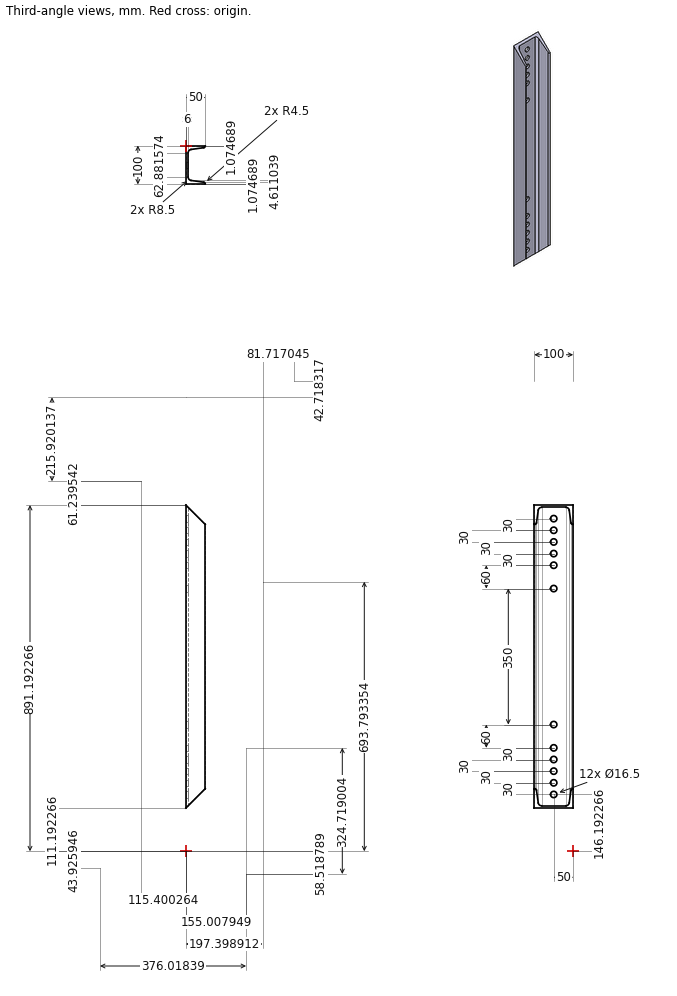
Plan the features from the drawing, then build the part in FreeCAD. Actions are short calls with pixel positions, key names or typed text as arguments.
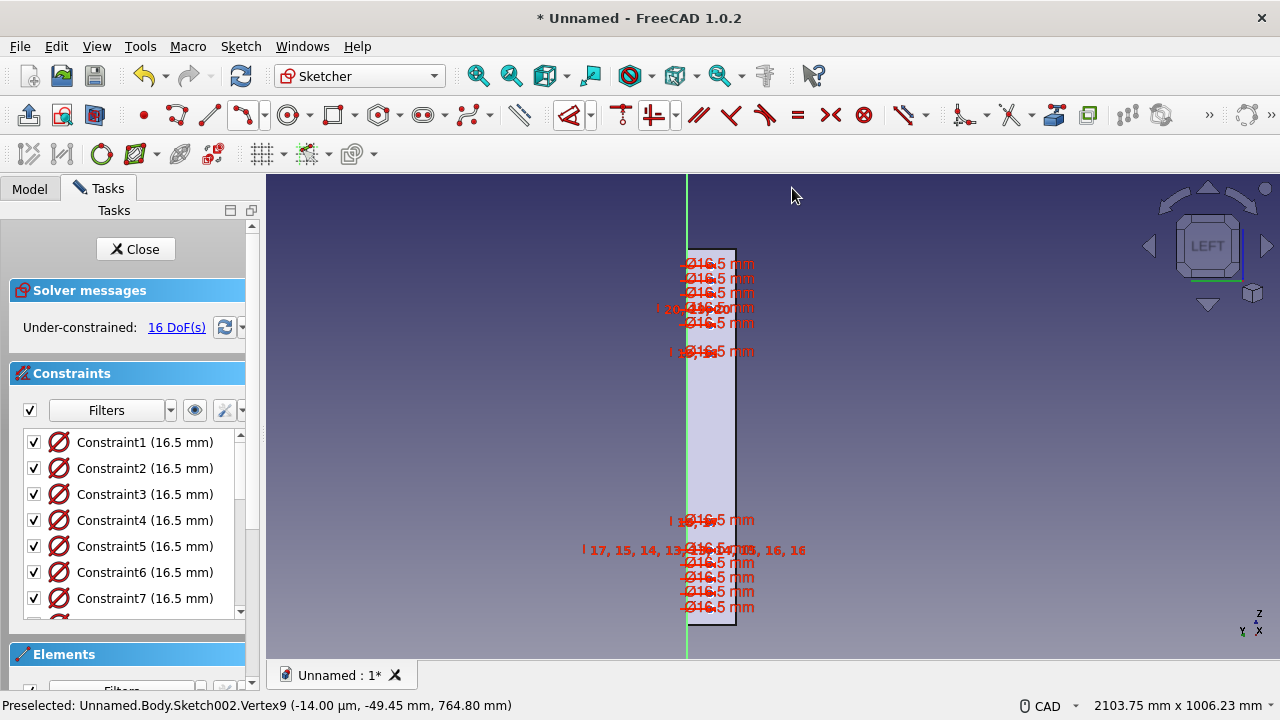
scroll(711, 310, up, 4)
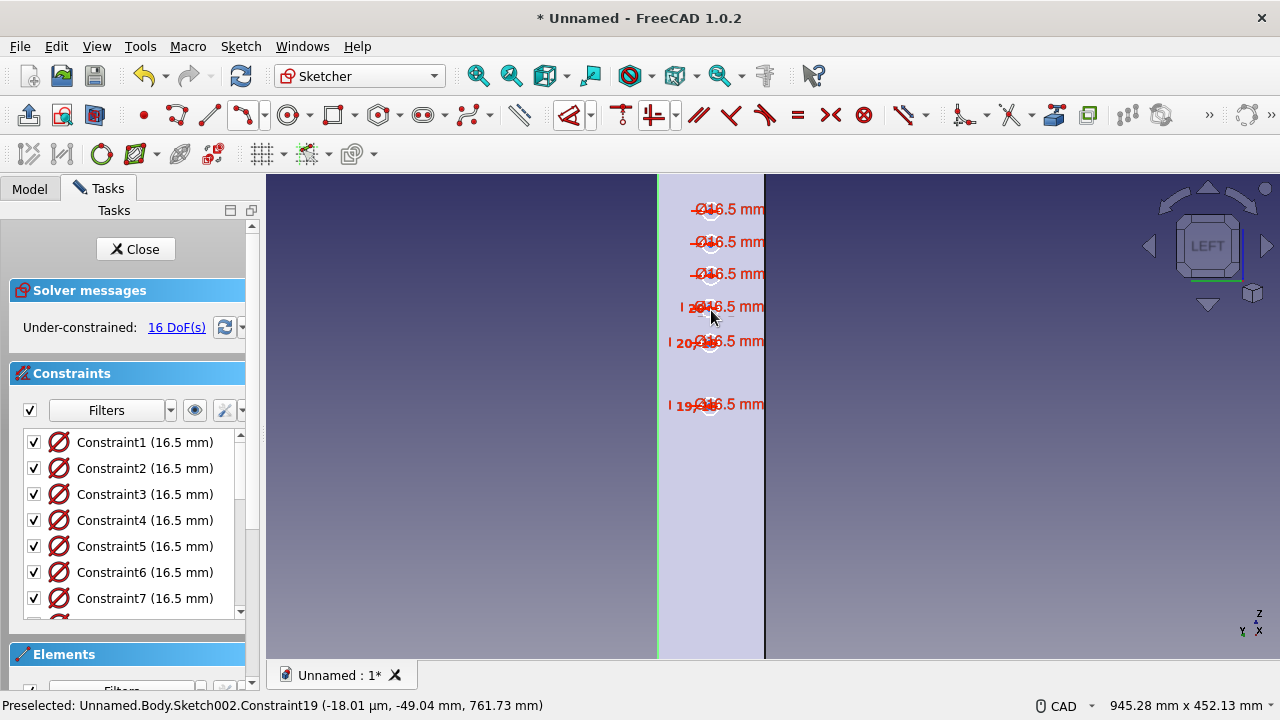
click(710, 309)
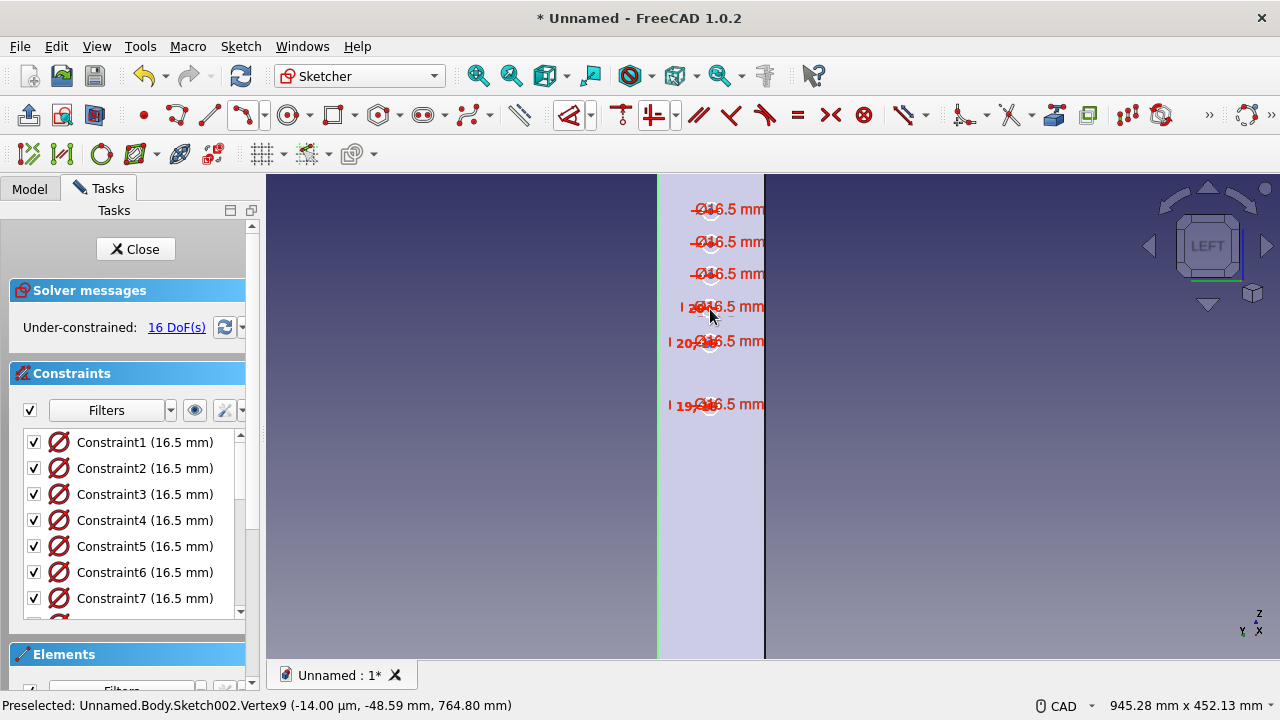
click(711, 276)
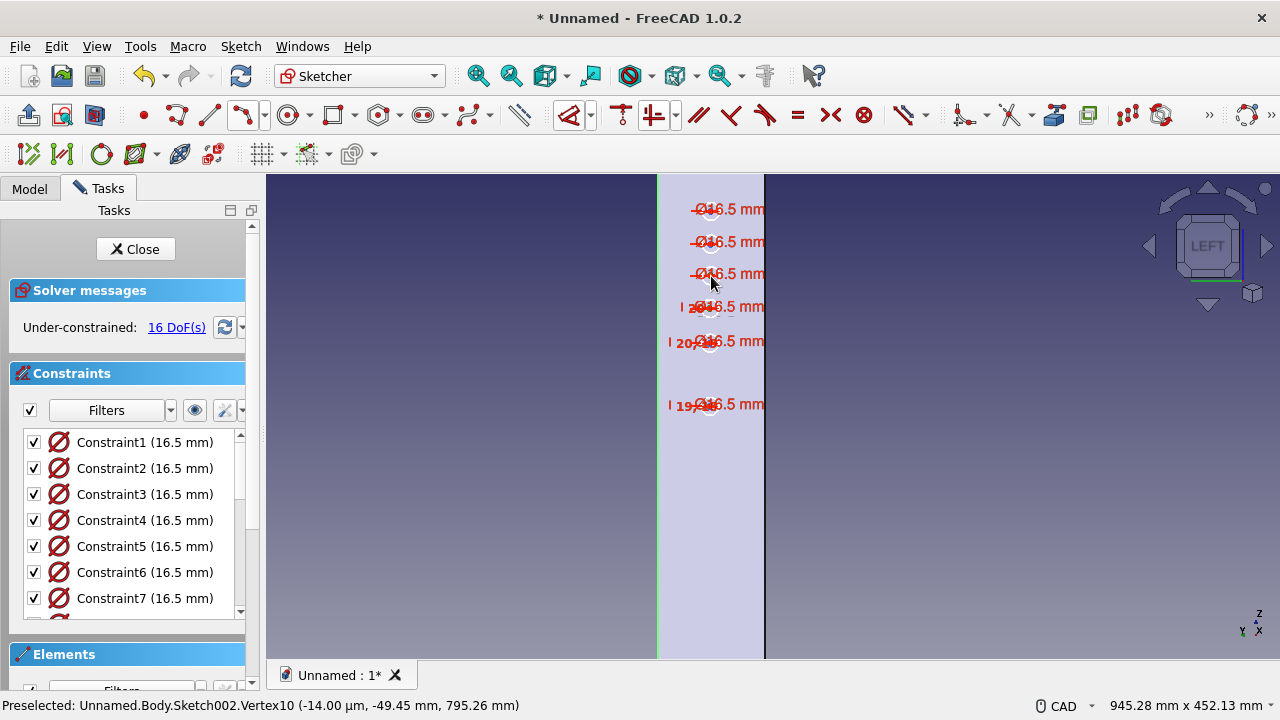
click(676, 116)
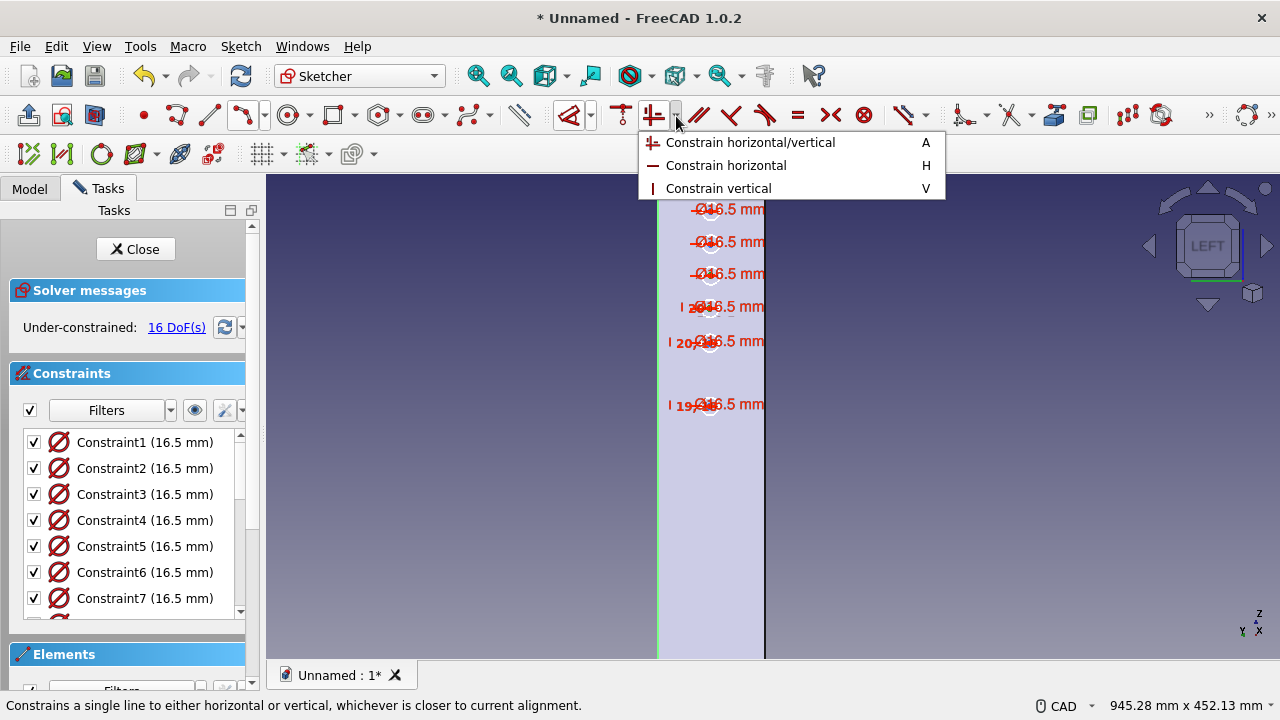
click(792, 188)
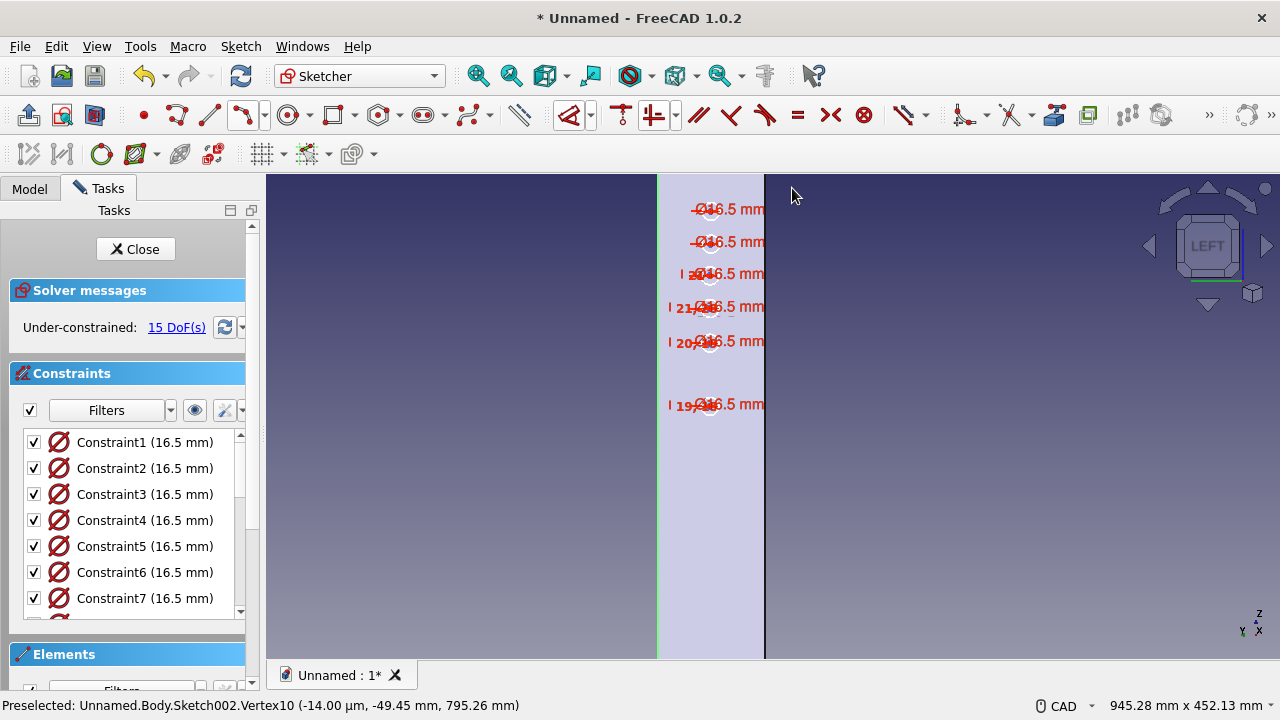
click(710, 276)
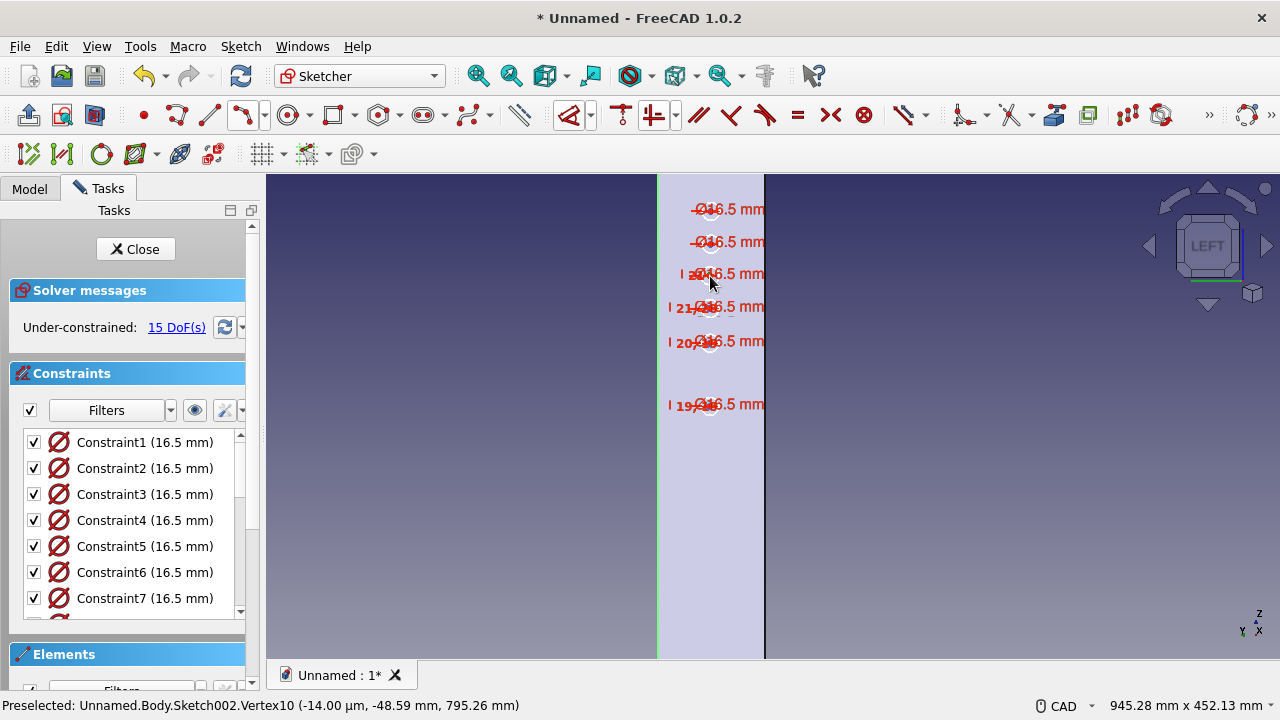
click(711, 244)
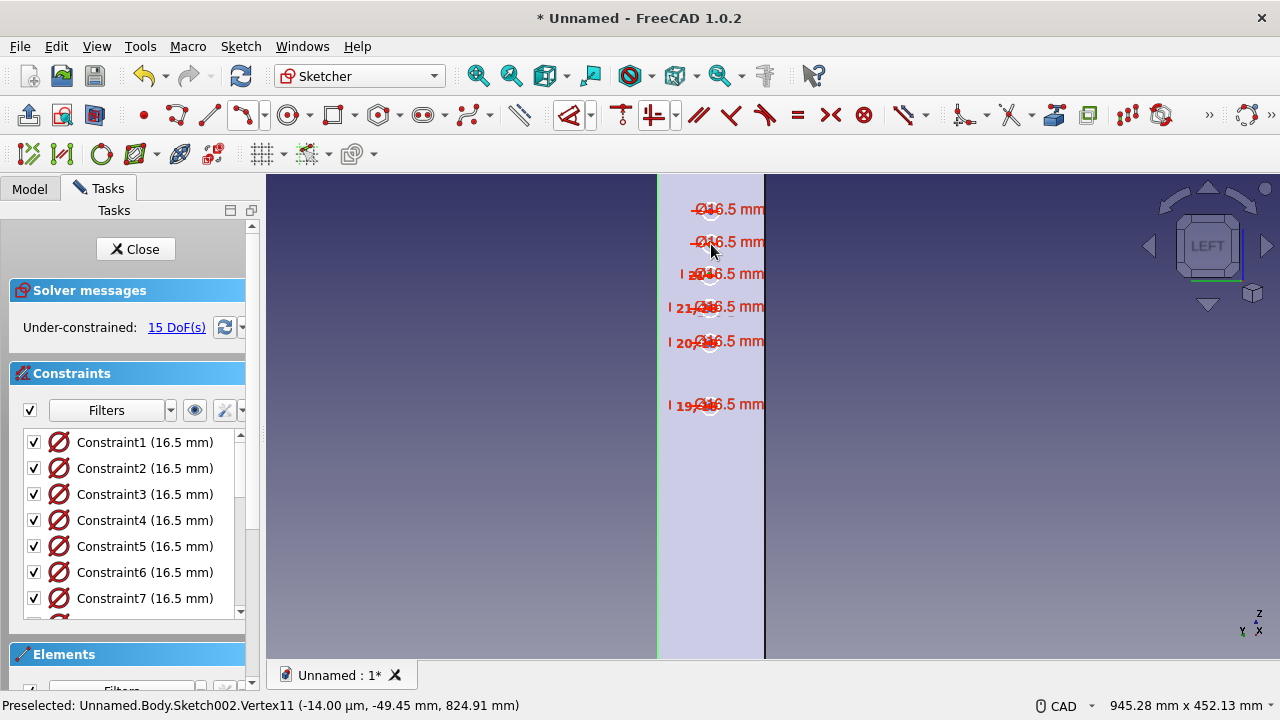
click(676, 116)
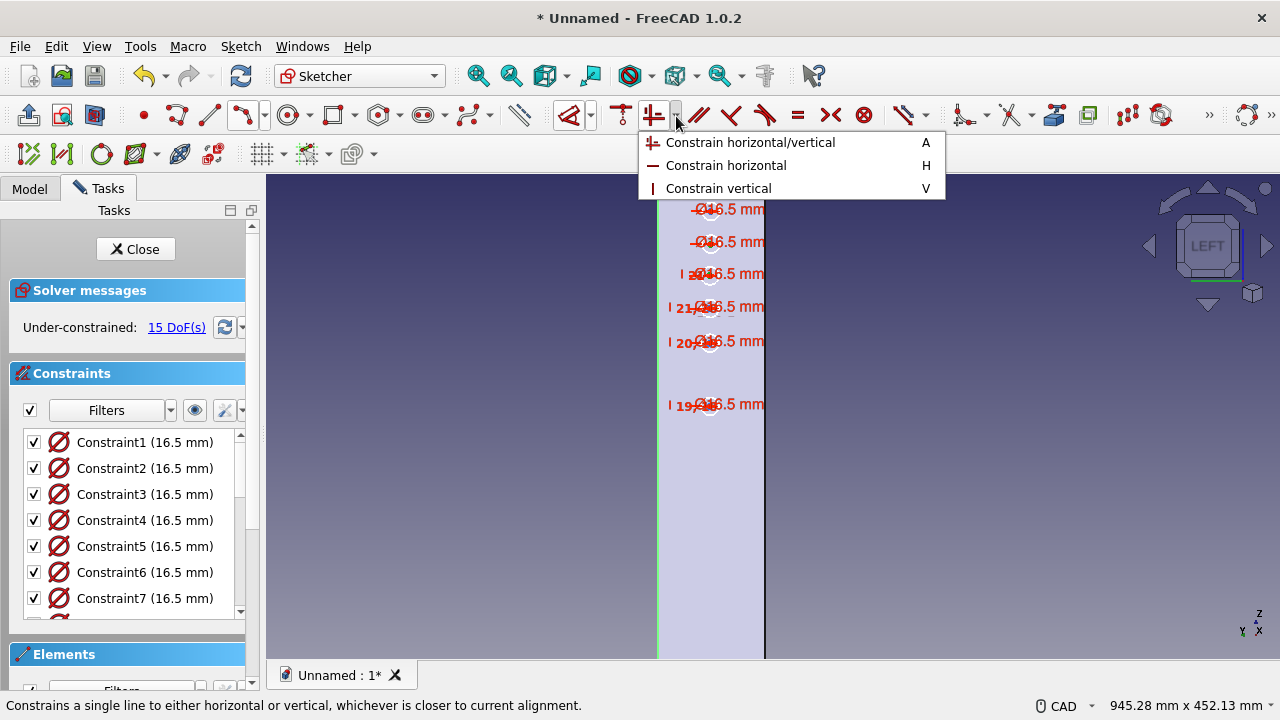
click(792, 188)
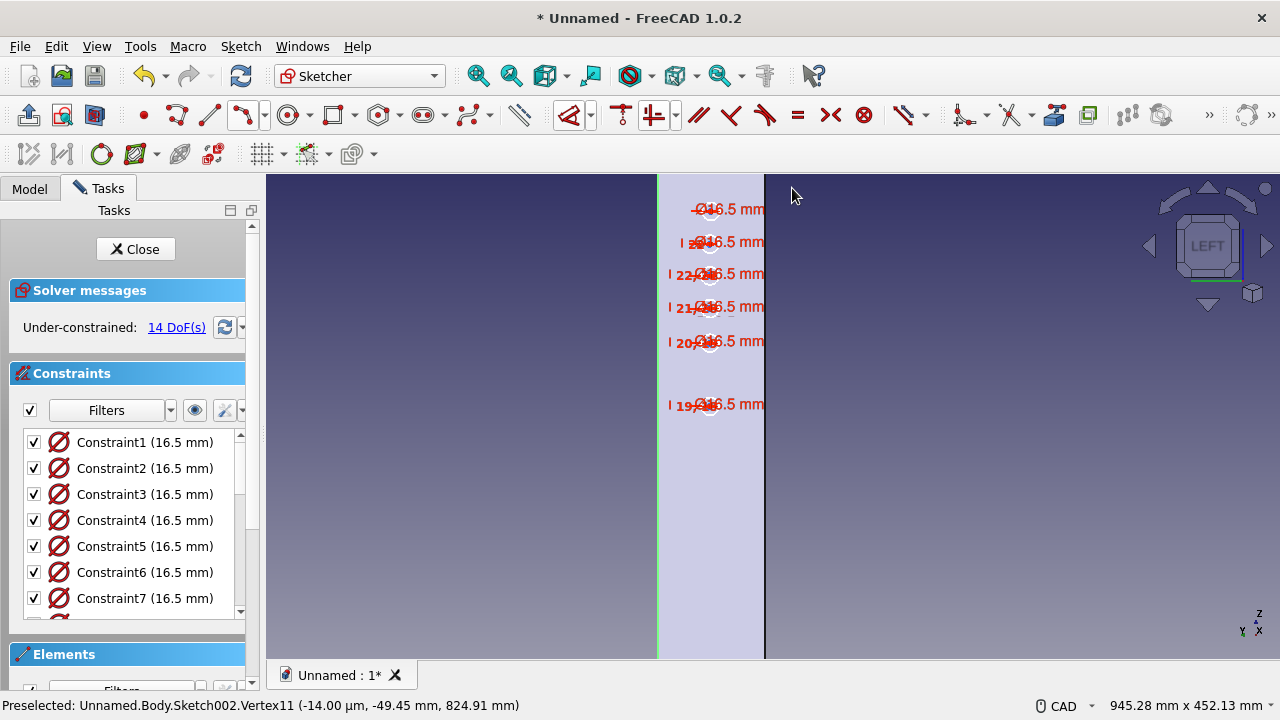
click(710, 244)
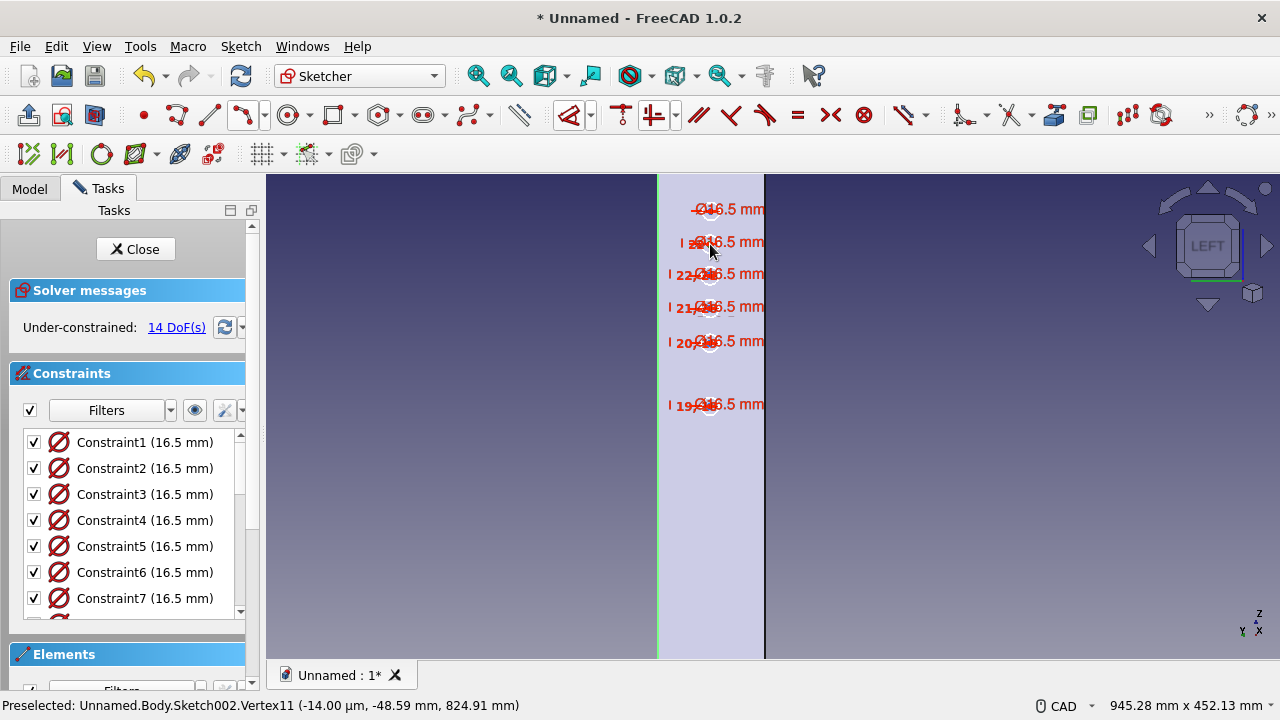
click(711, 211)